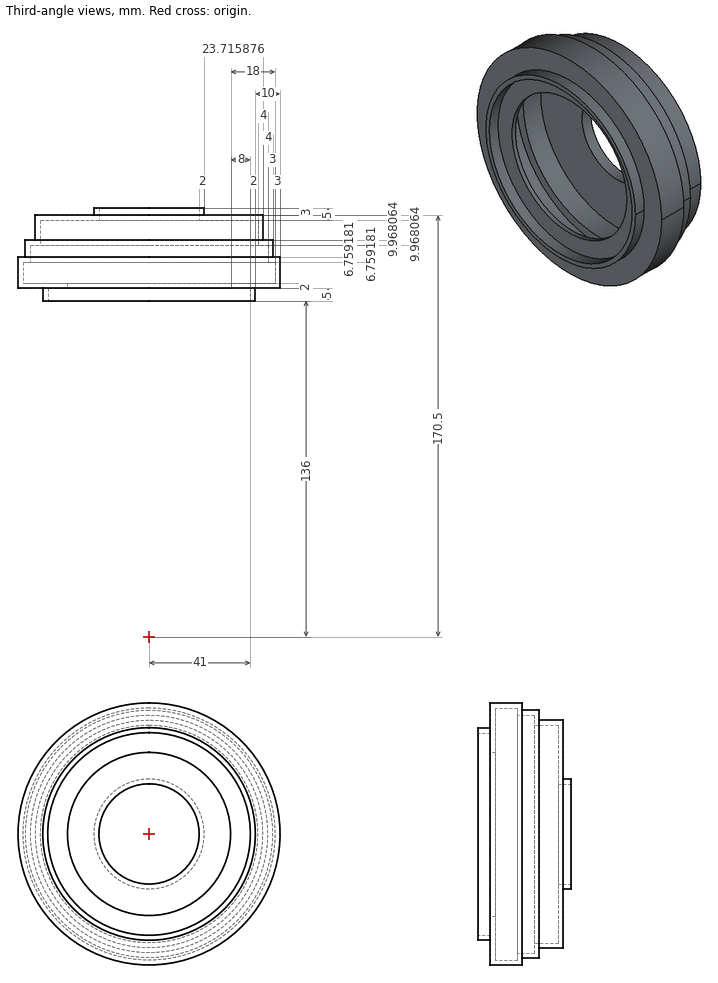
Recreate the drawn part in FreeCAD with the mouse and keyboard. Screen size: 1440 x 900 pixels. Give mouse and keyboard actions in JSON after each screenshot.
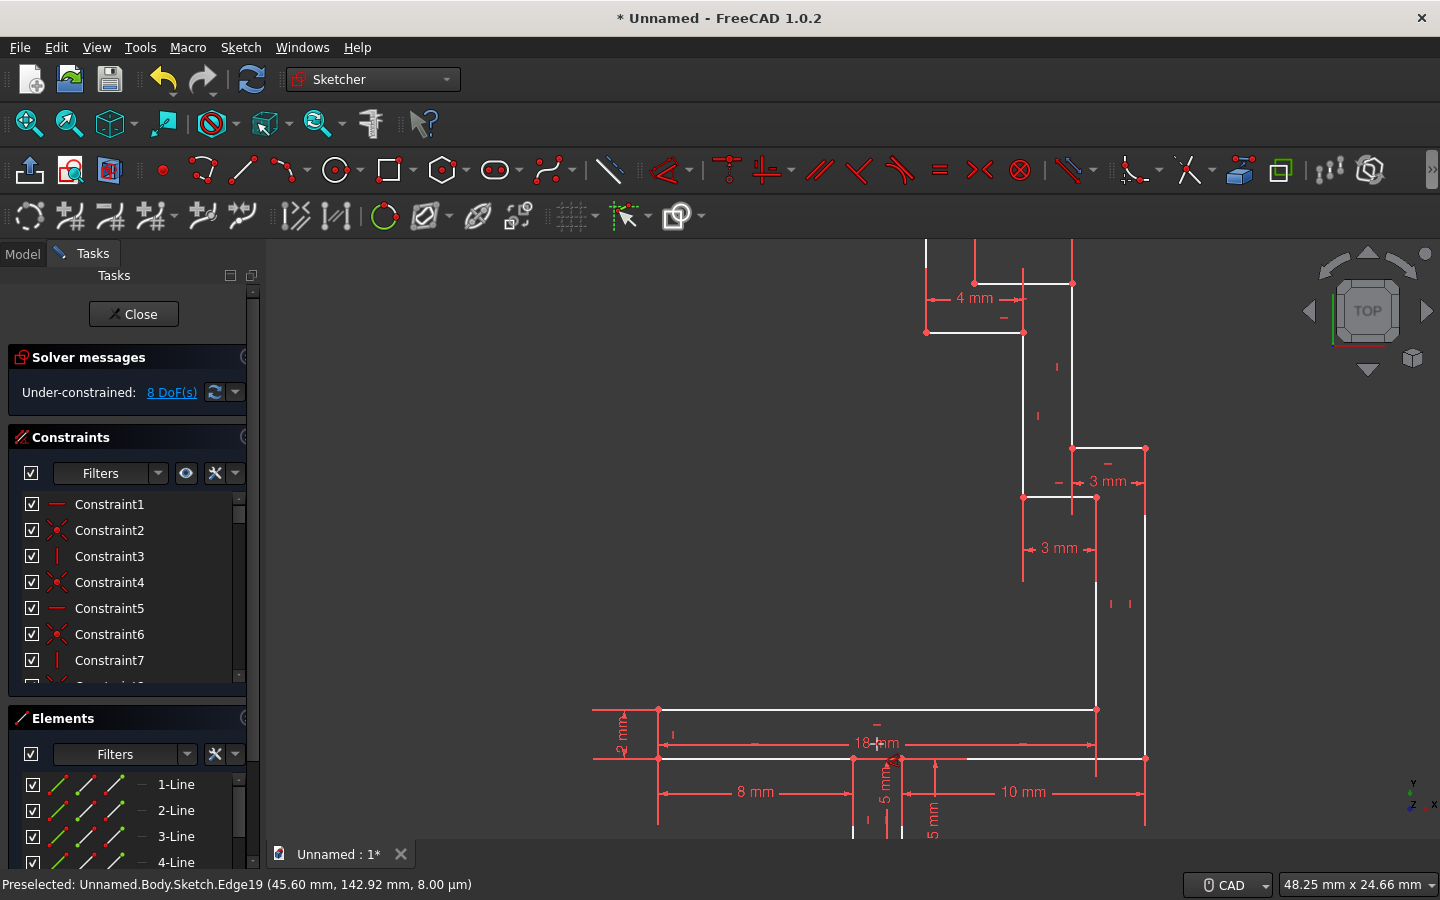
{"action": "scroll", "coordinate": [815, 634], "scroll_direction": "down", "scroll_amount": 4}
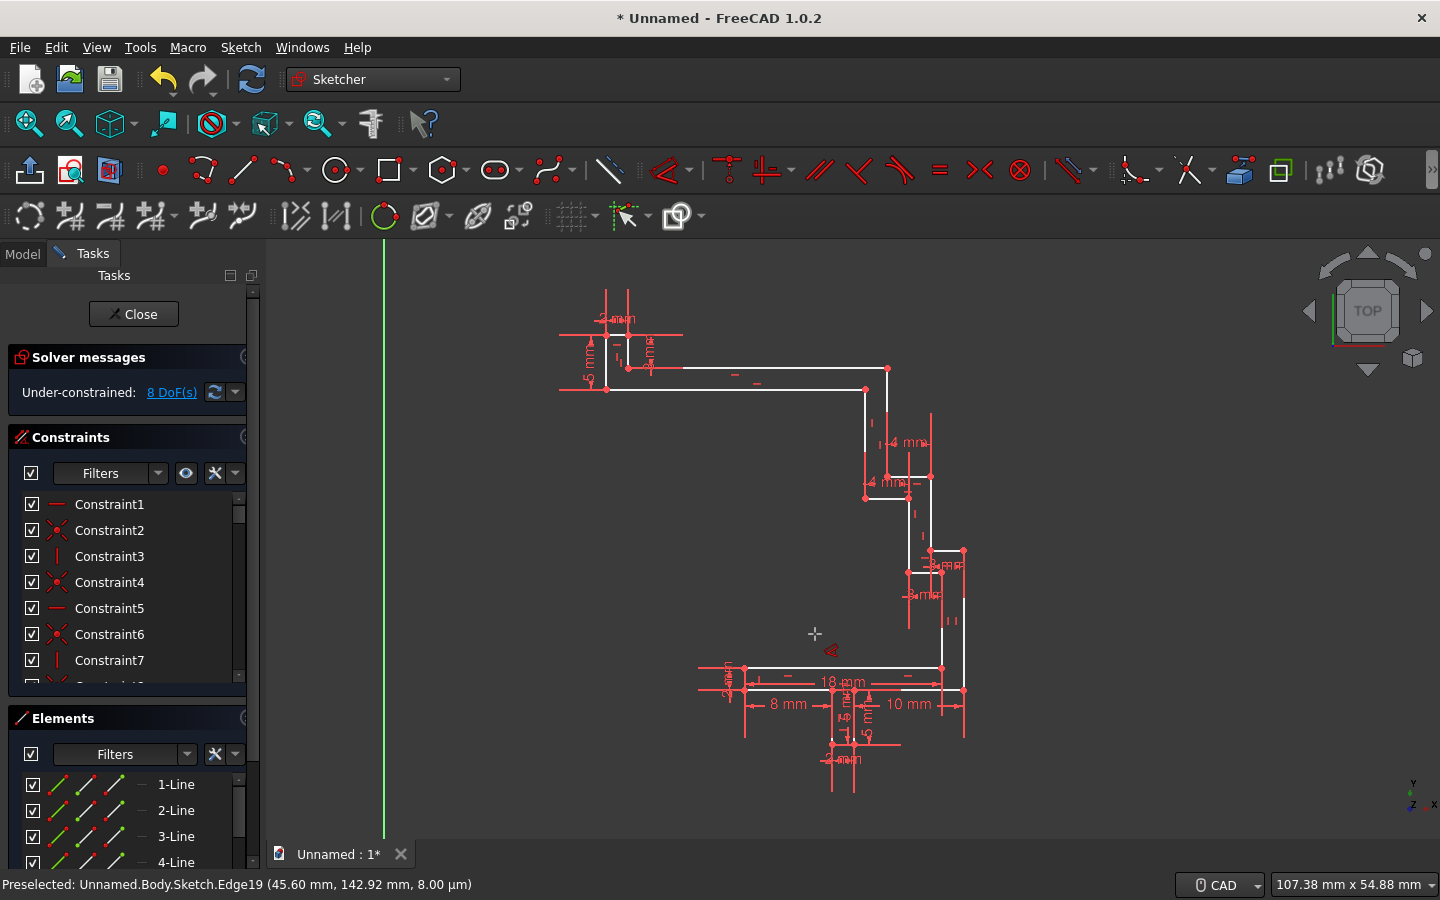
{"action": "left_click", "coordinate": [832, 745]}
{"action": "left_click", "coordinate": [608, 711]}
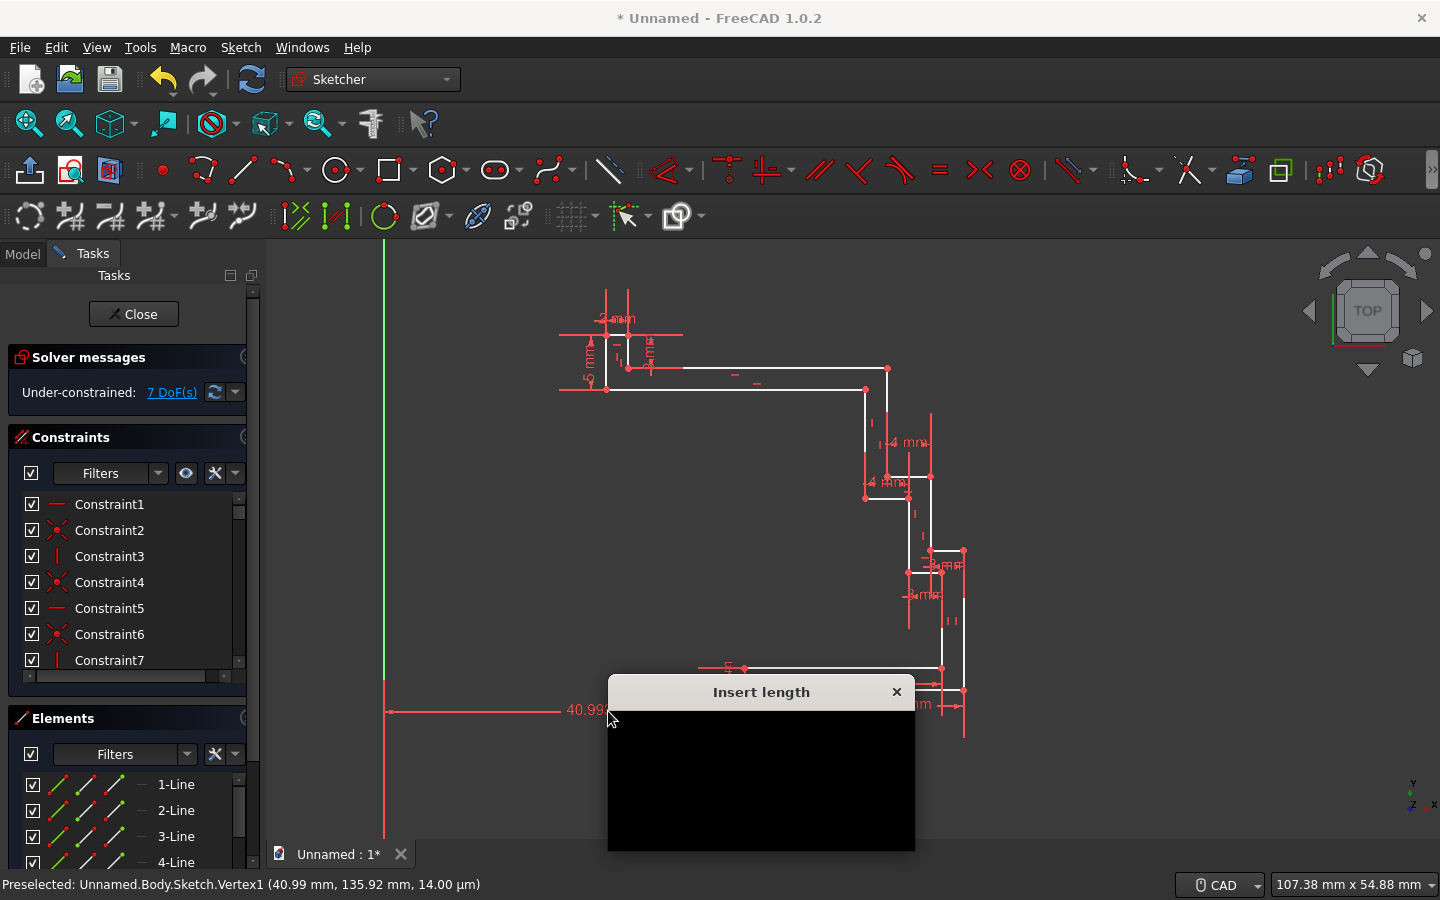
{"action": "type", "text": "41"}
{"action": "key", "text": "Return"}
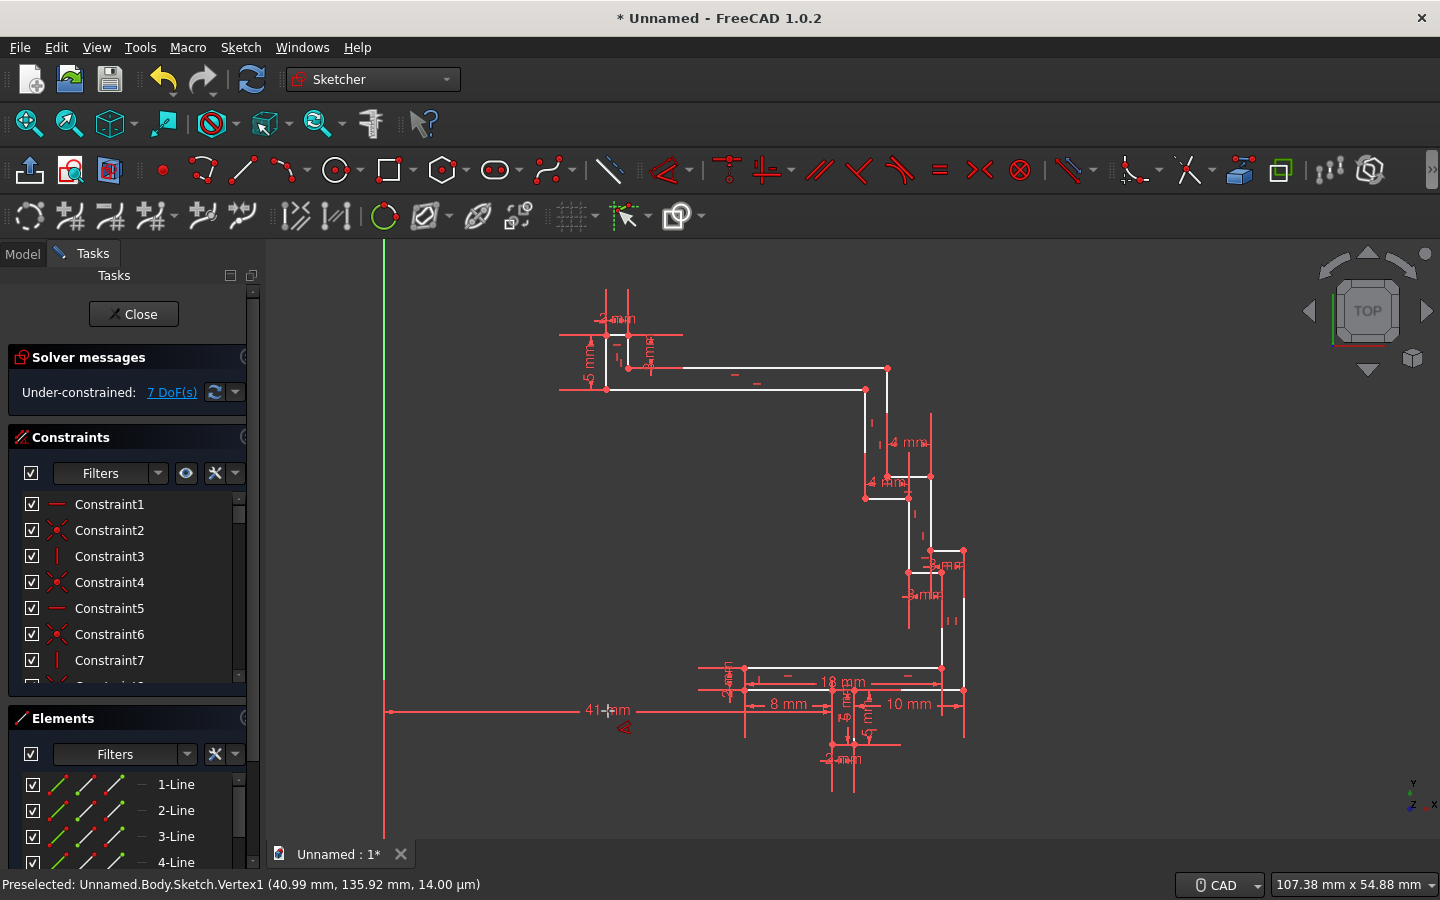
{"action": "left_click", "coordinate": [832, 745]}
{"action": "left_click", "coordinate": [350, 778]}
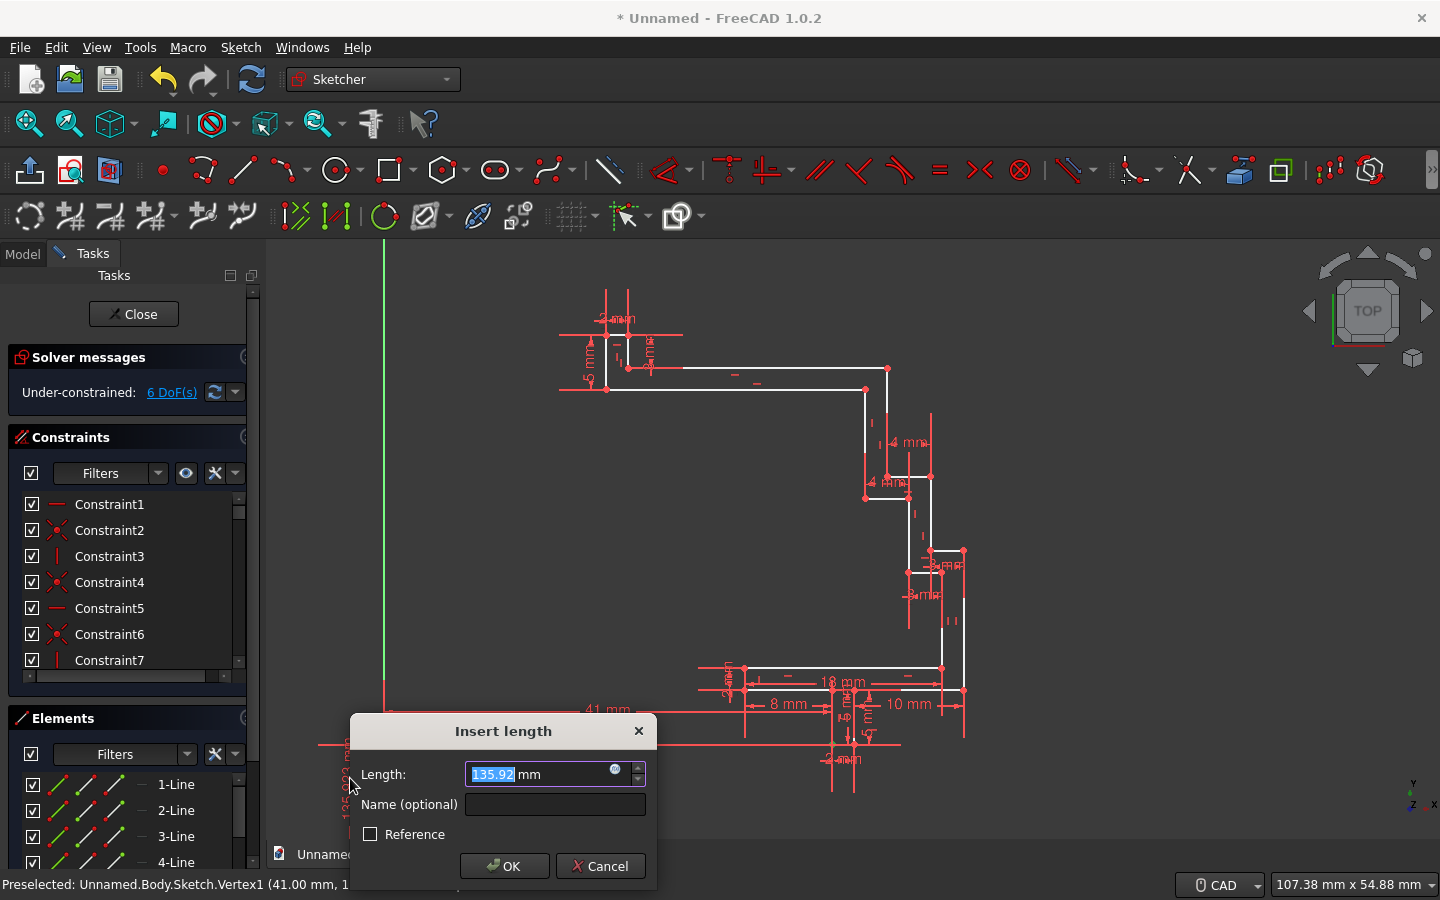
{"action": "type", "text": "136"}
{"action": "key", "text": "Return"}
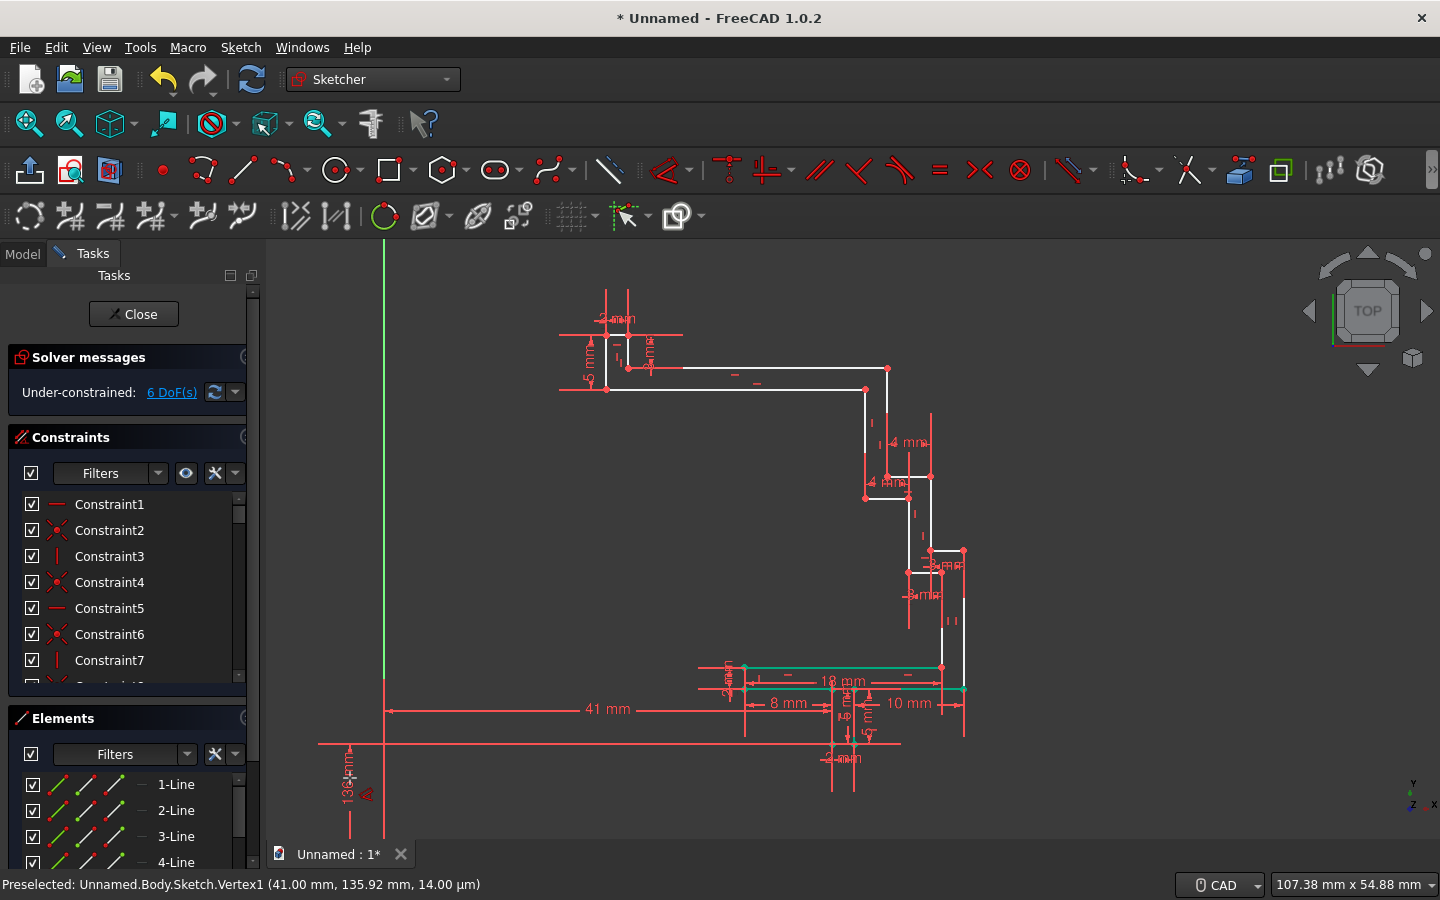
{"action": "left_click", "coordinate": [887, 368]}
{"action": "left_click", "coordinate": [350, 590]}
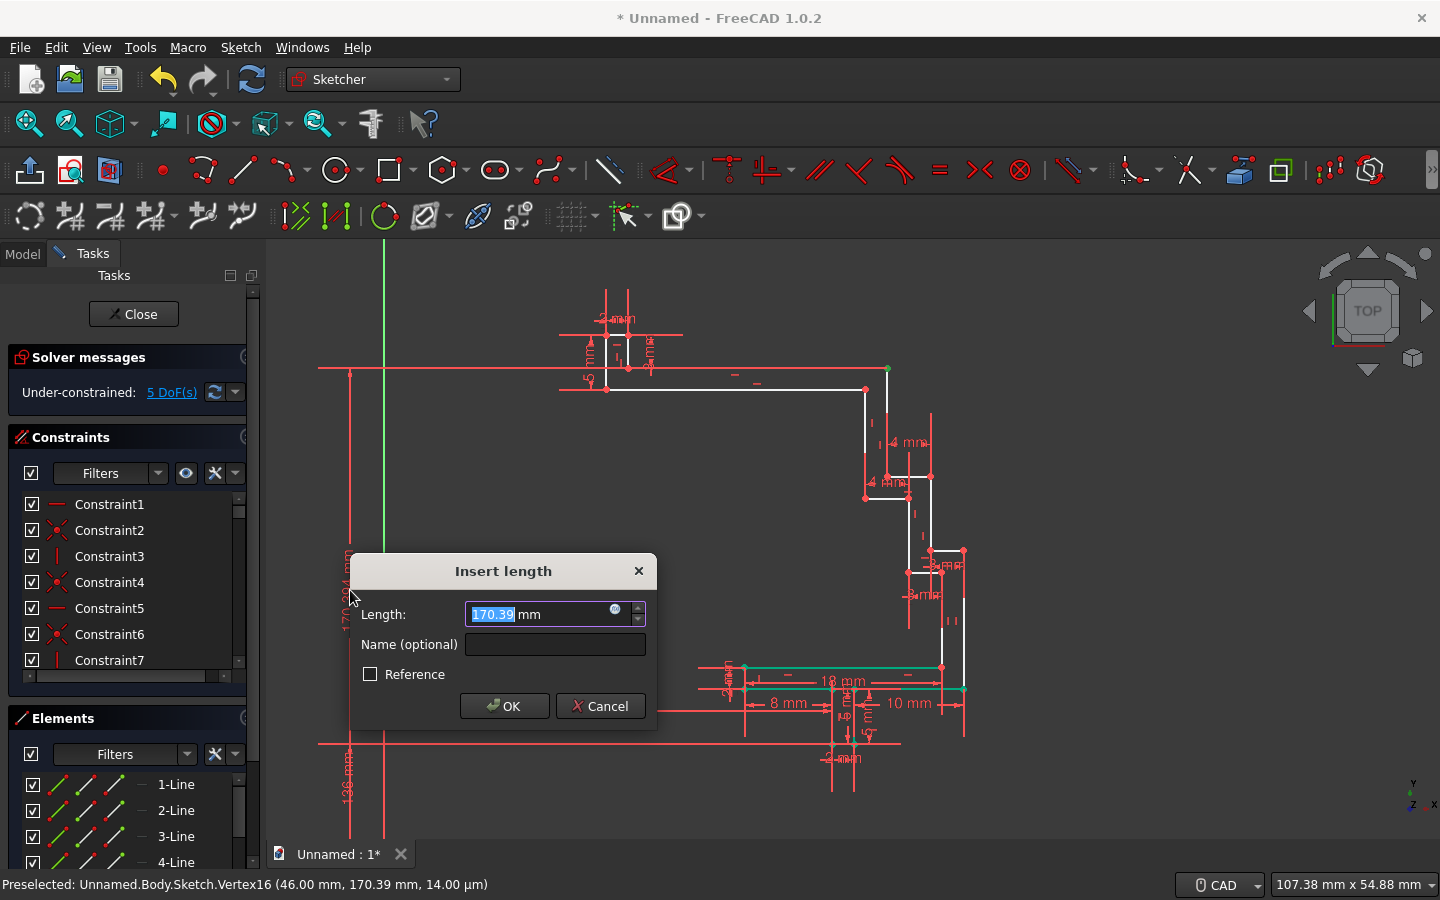
{"action": "type", "text": "170.5"}
{"action": "key", "text": "Return"}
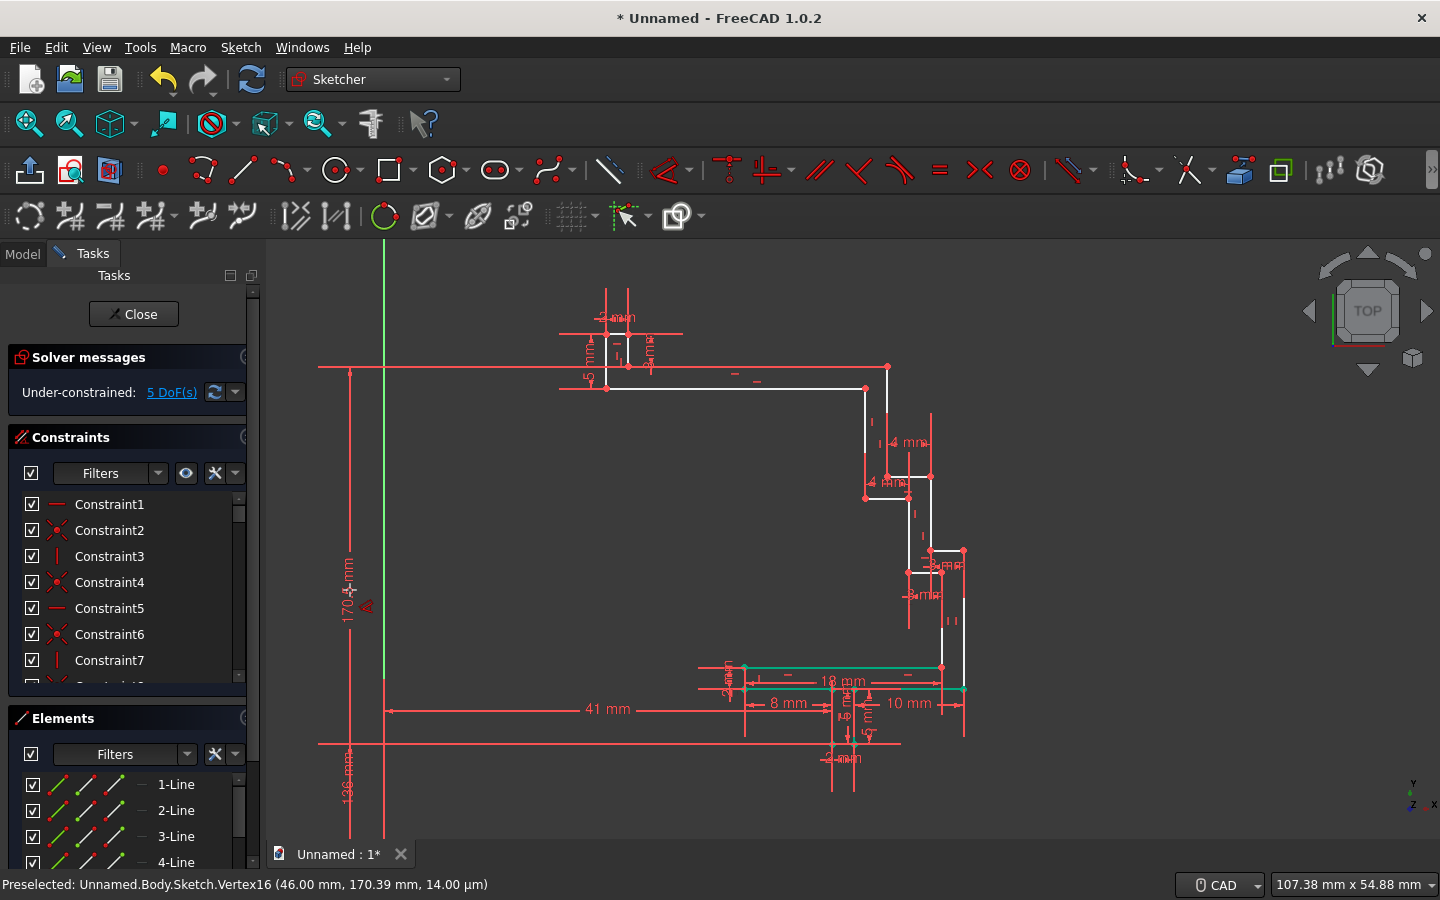
{"action": "left_click", "coordinate": [931, 529]}
{"action": "left_click", "coordinate": [965, 514]}